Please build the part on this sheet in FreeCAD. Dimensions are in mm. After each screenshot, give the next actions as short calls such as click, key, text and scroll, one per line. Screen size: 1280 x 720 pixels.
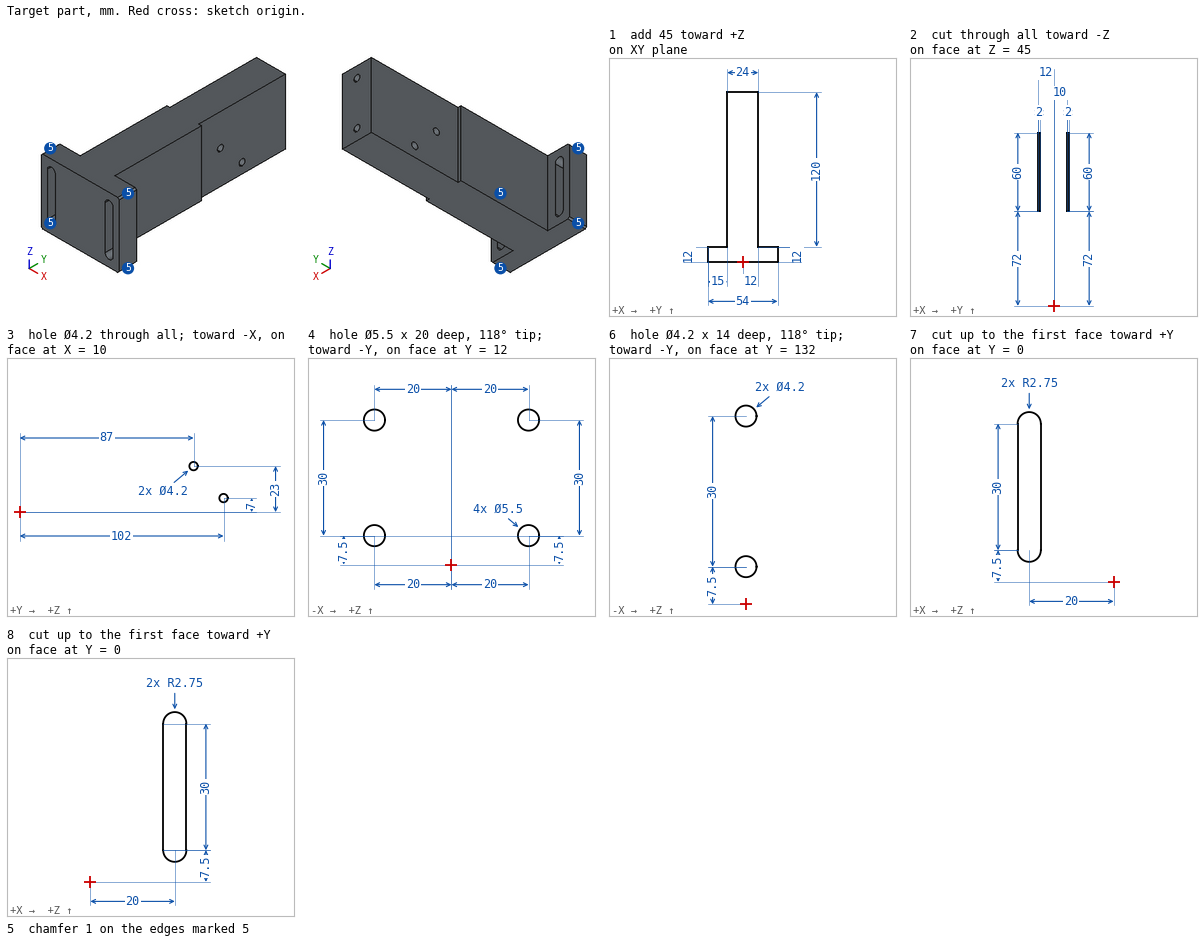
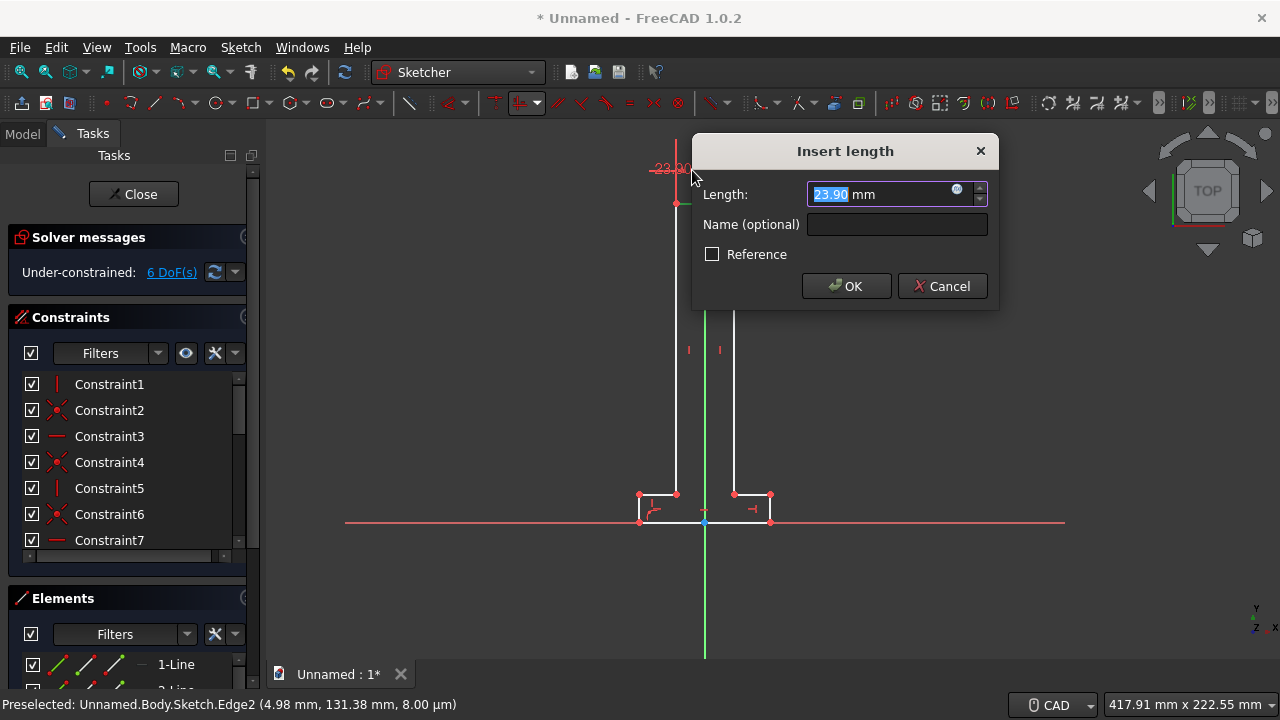
text(24)
key(Return)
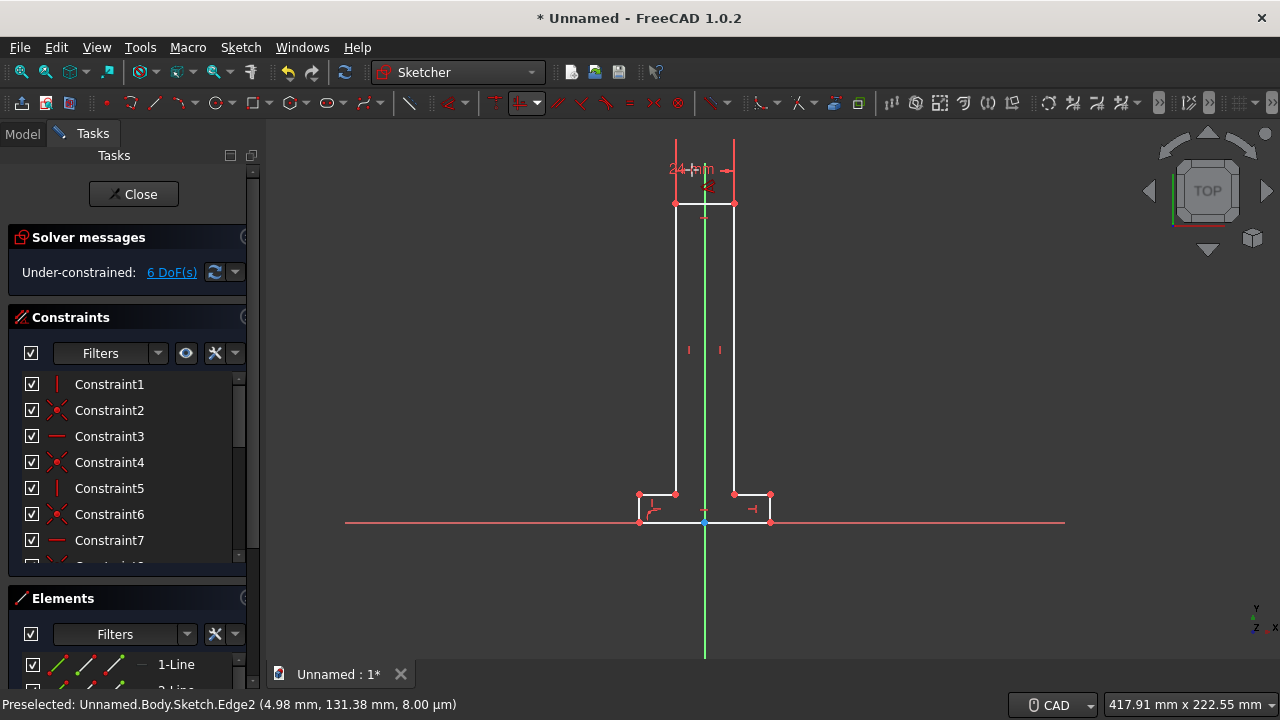
scroll(665, 495, up, 2)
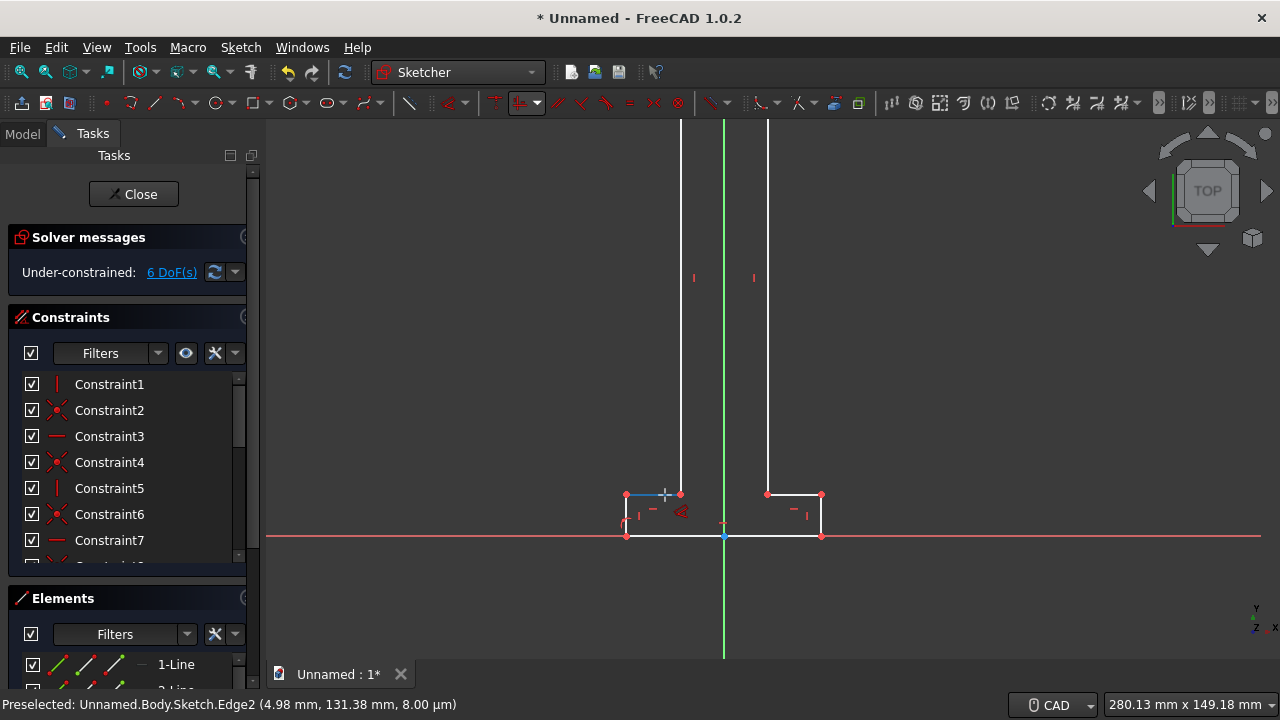
click(664, 495)
click(653, 461)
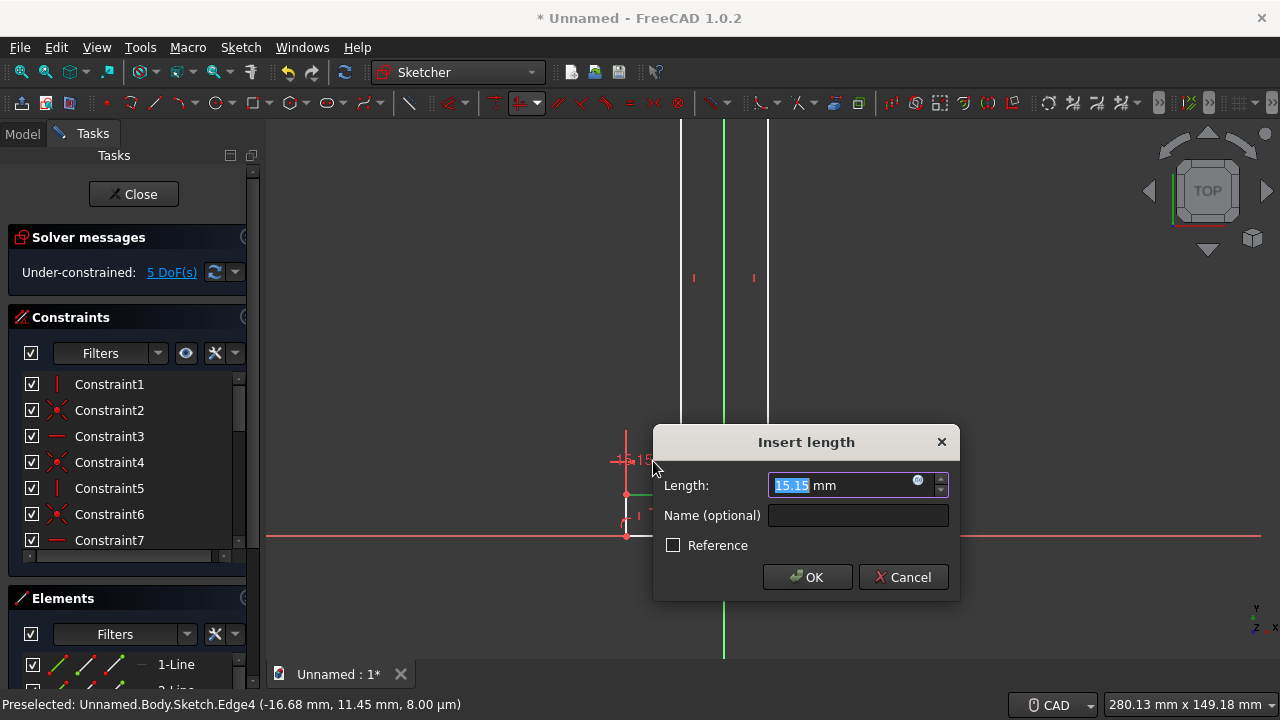
text(15)
key(Return)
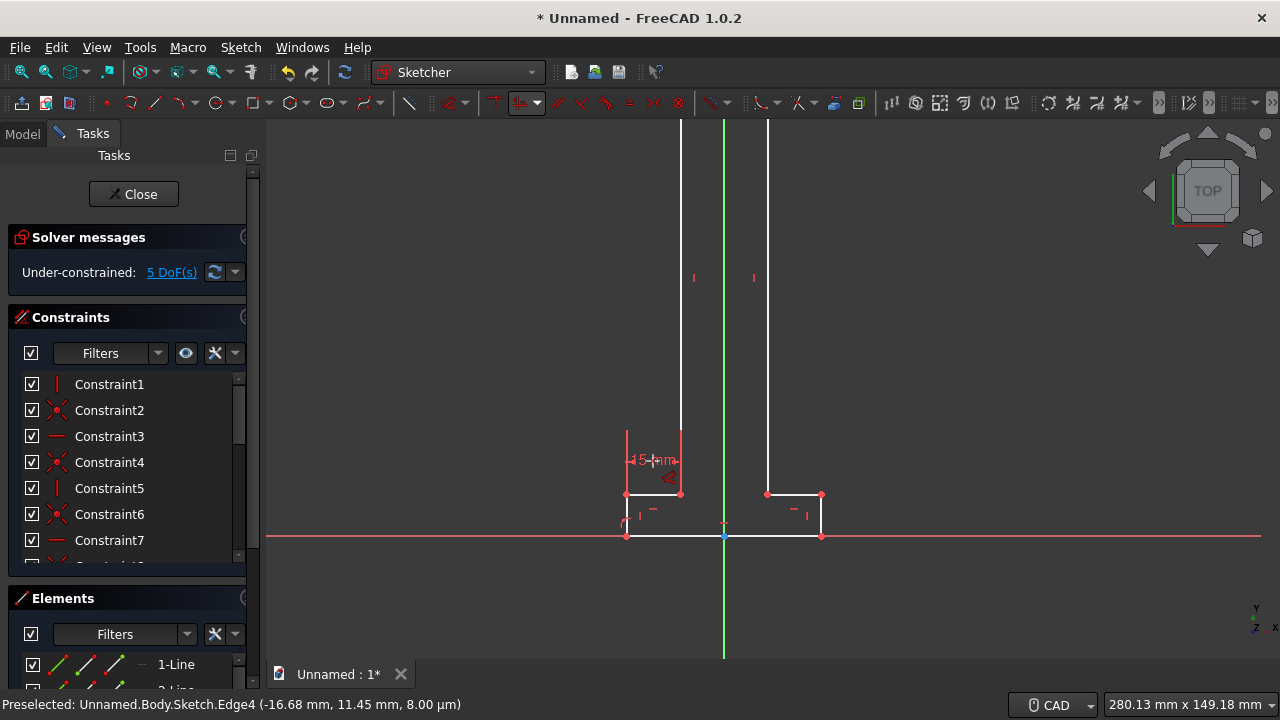
click(627, 507)
click(593, 515)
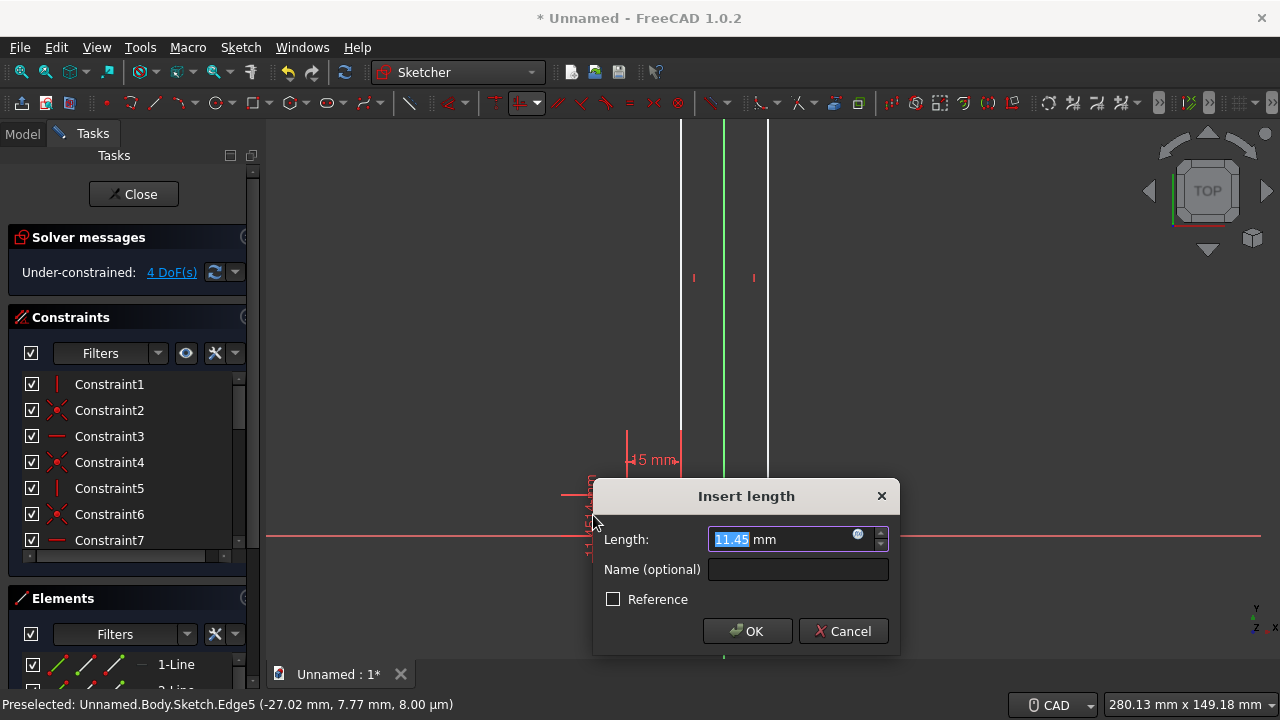
text(12)
key(Return)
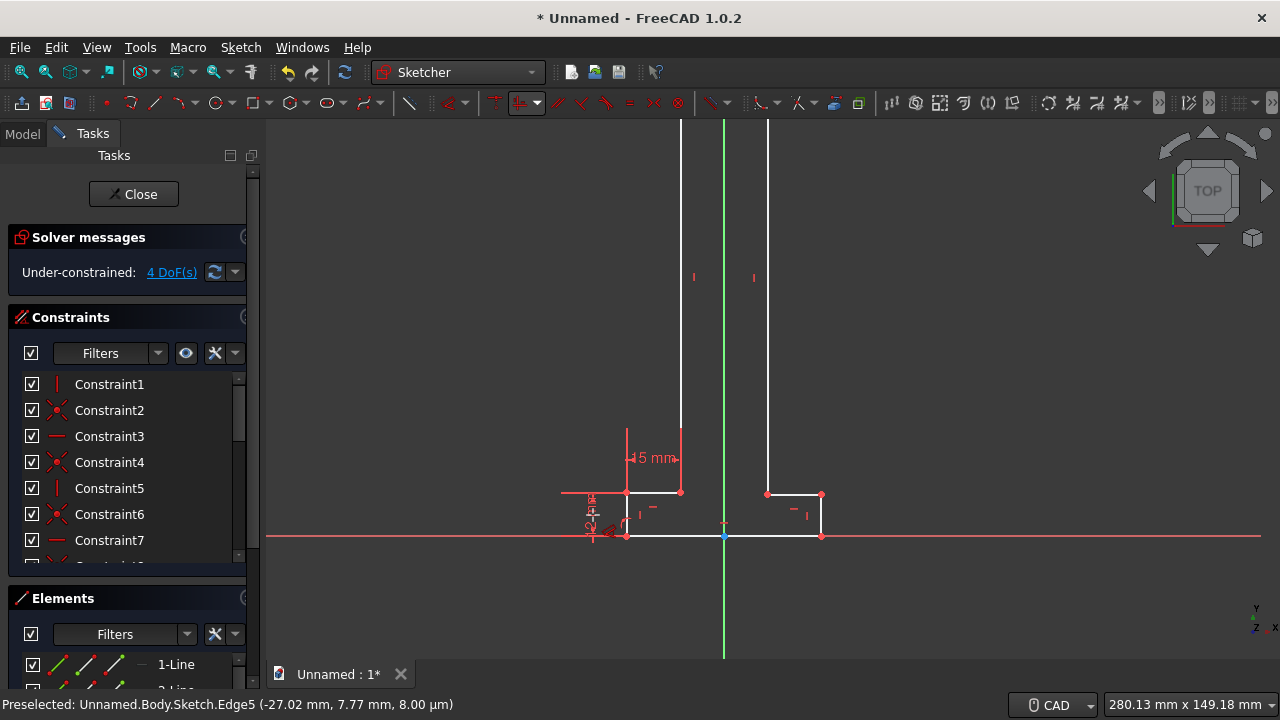
click(685, 536)
click(679, 570)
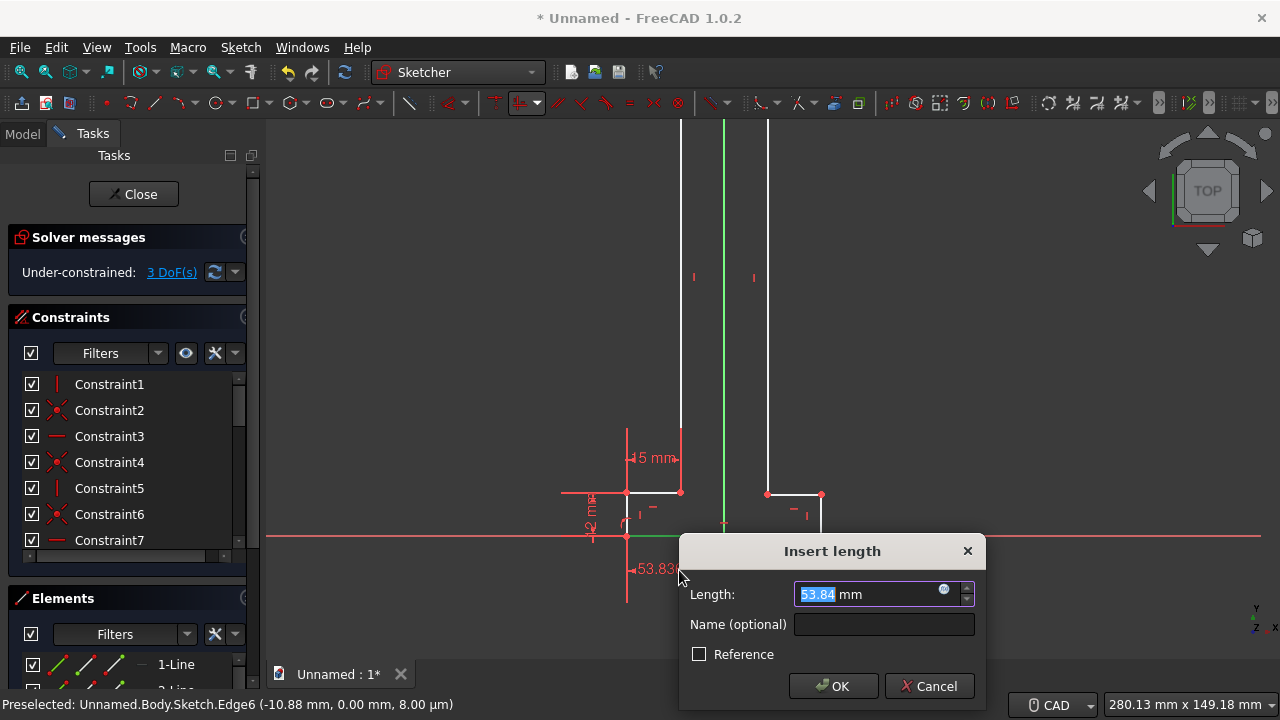
text(54)
key(Return)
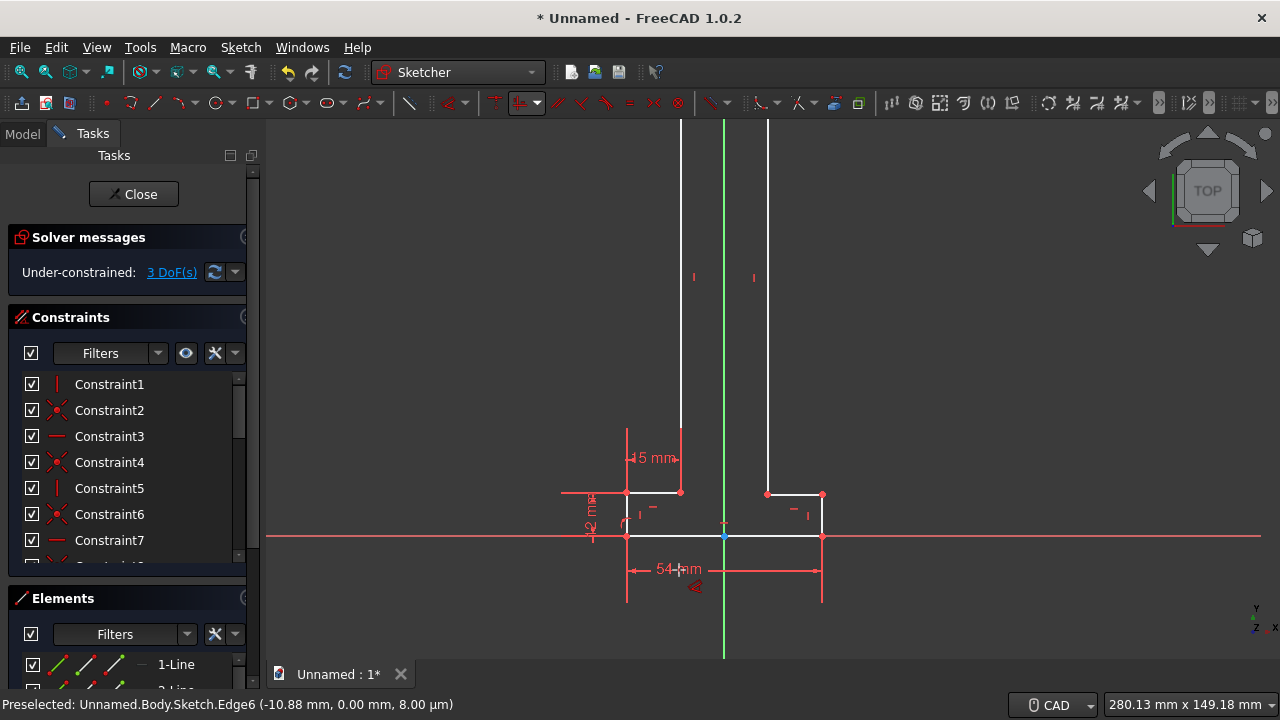
click(822, 524)
click(856, 515)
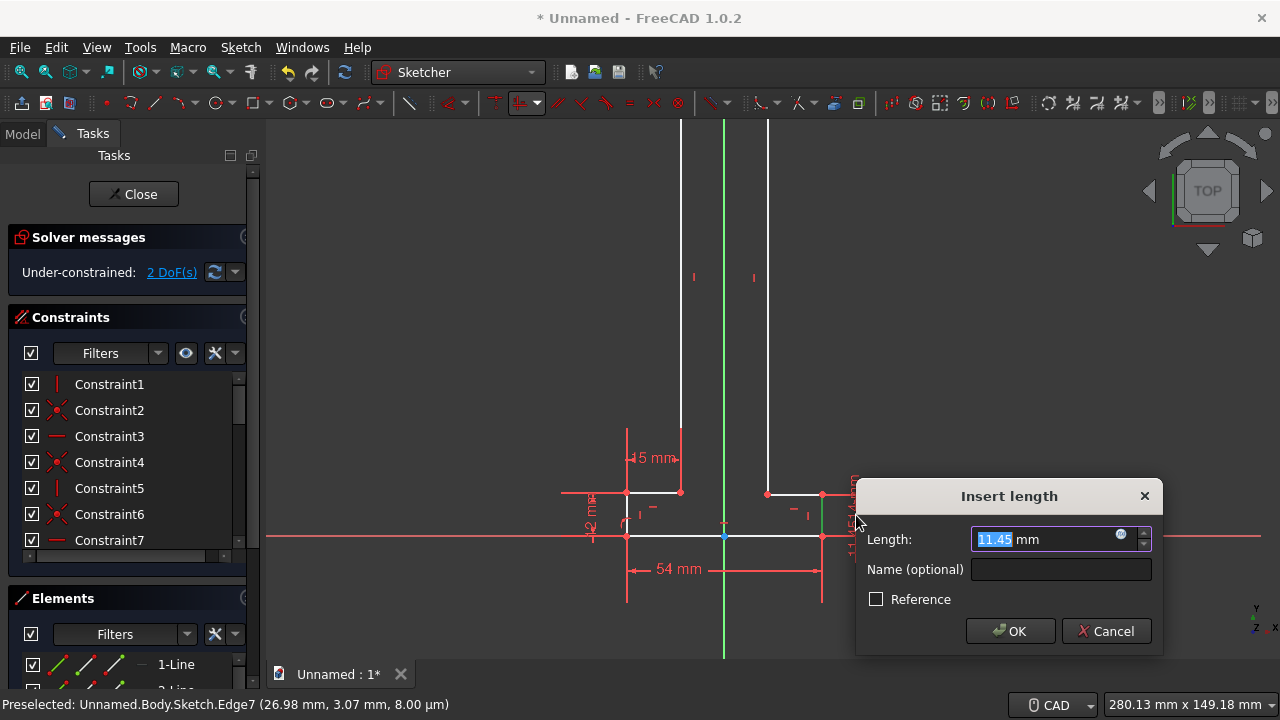
text(12)
key(Return)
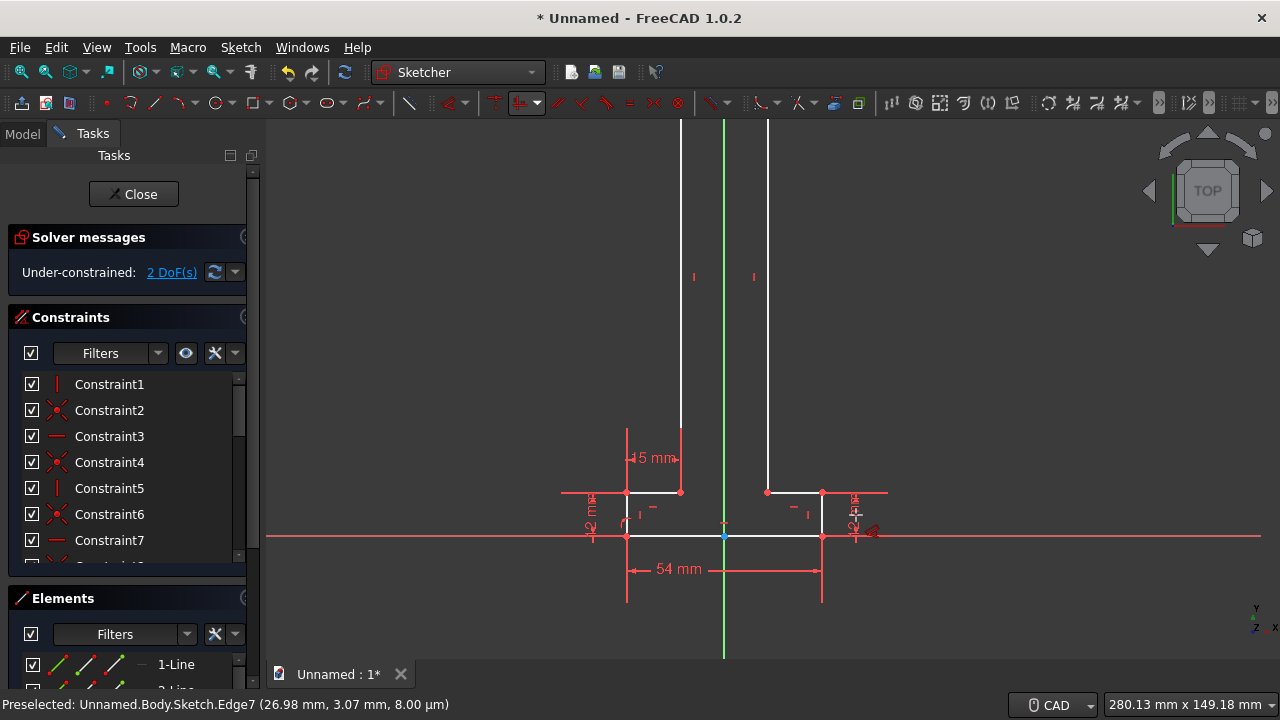
click(768, 363)
click(802, 320)